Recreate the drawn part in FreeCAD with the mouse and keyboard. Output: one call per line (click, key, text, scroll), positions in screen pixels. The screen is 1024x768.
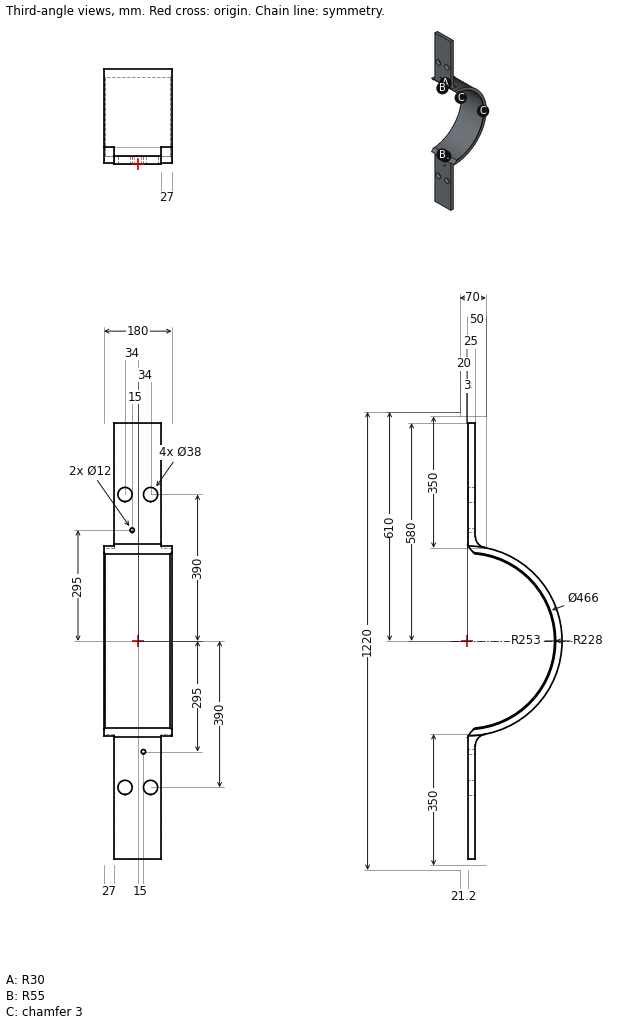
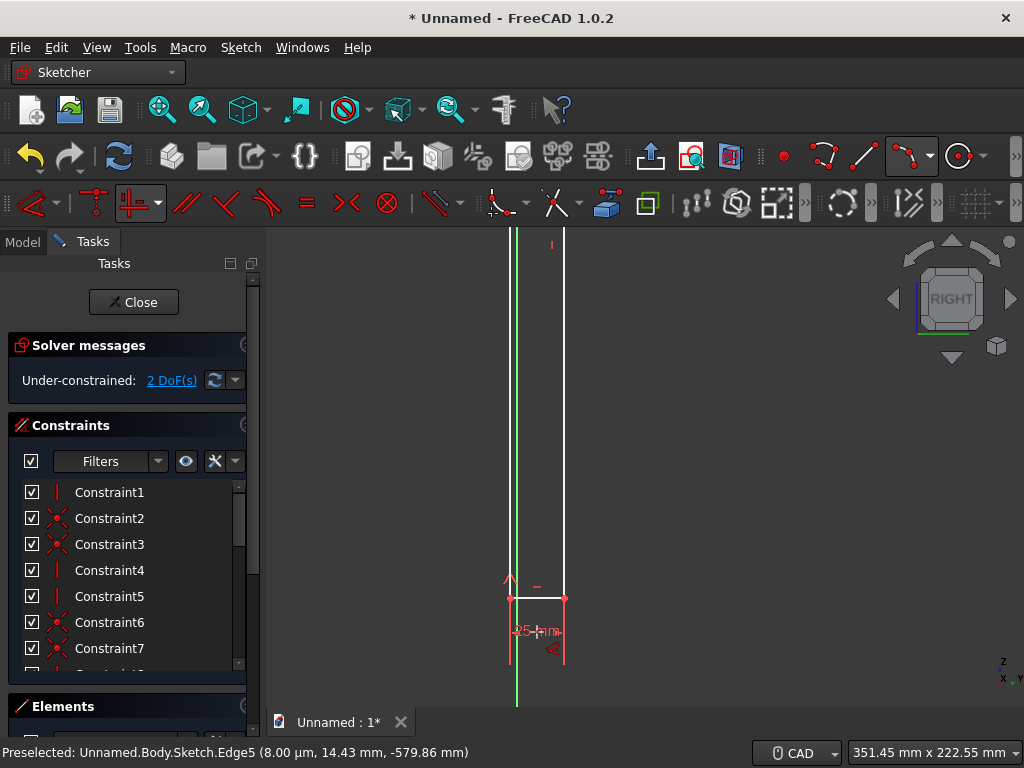
scroll(550, 606, down, 11)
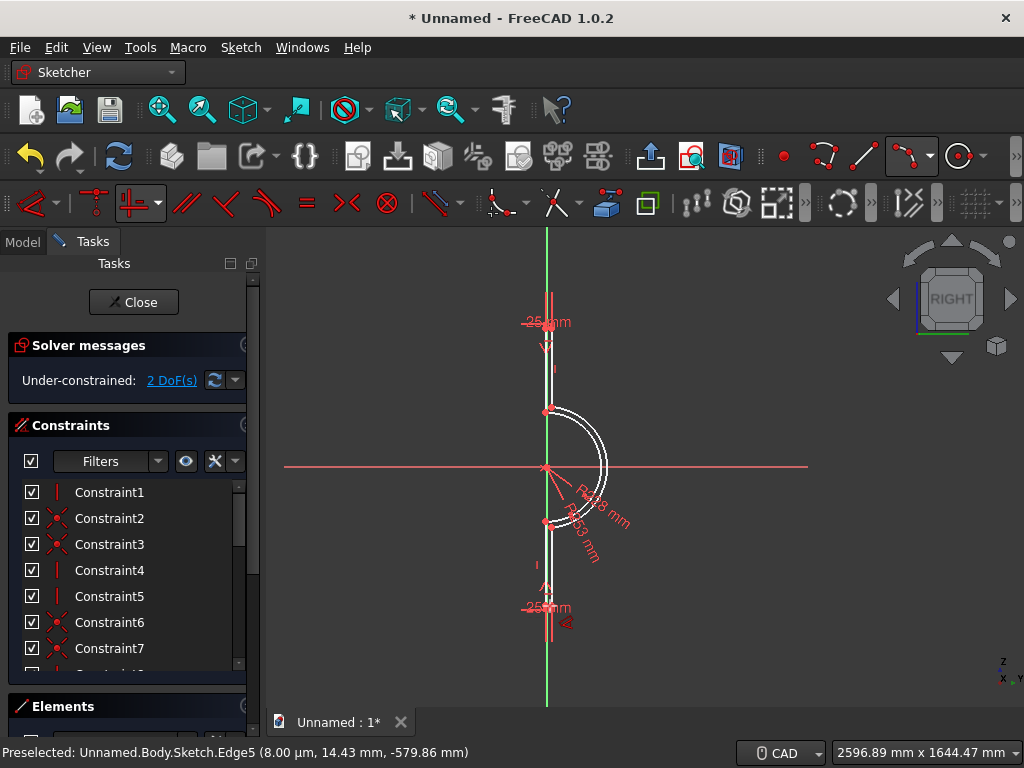
scroll(546, 329, up, 21)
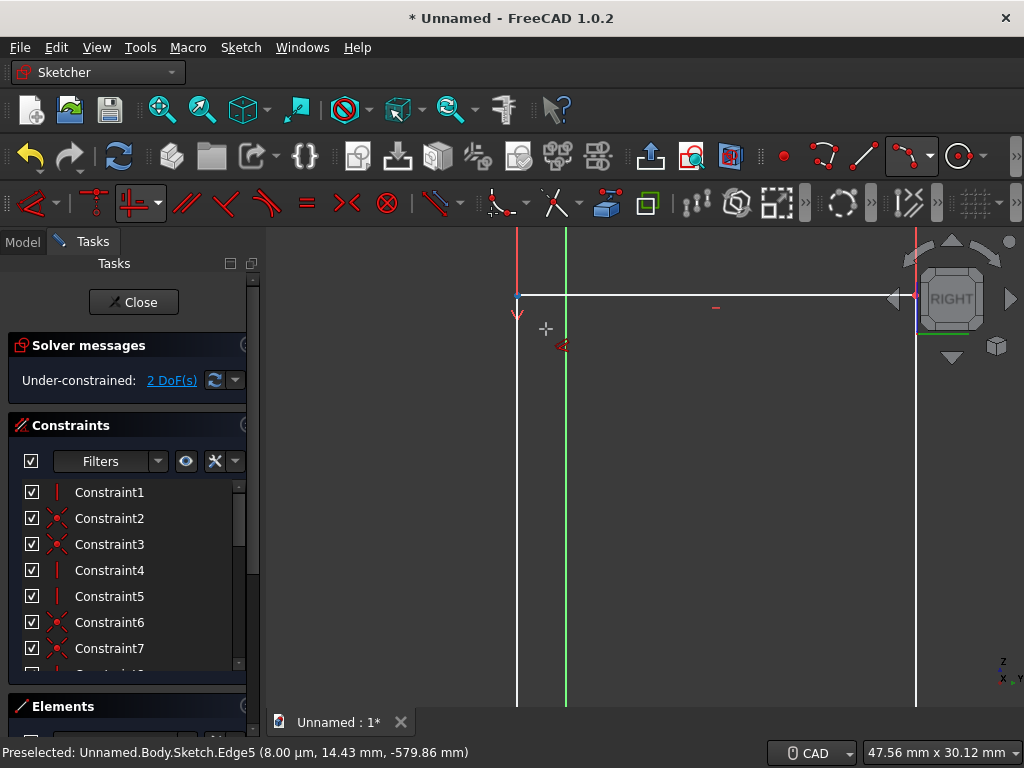
click(517, 295)
click(542, 261)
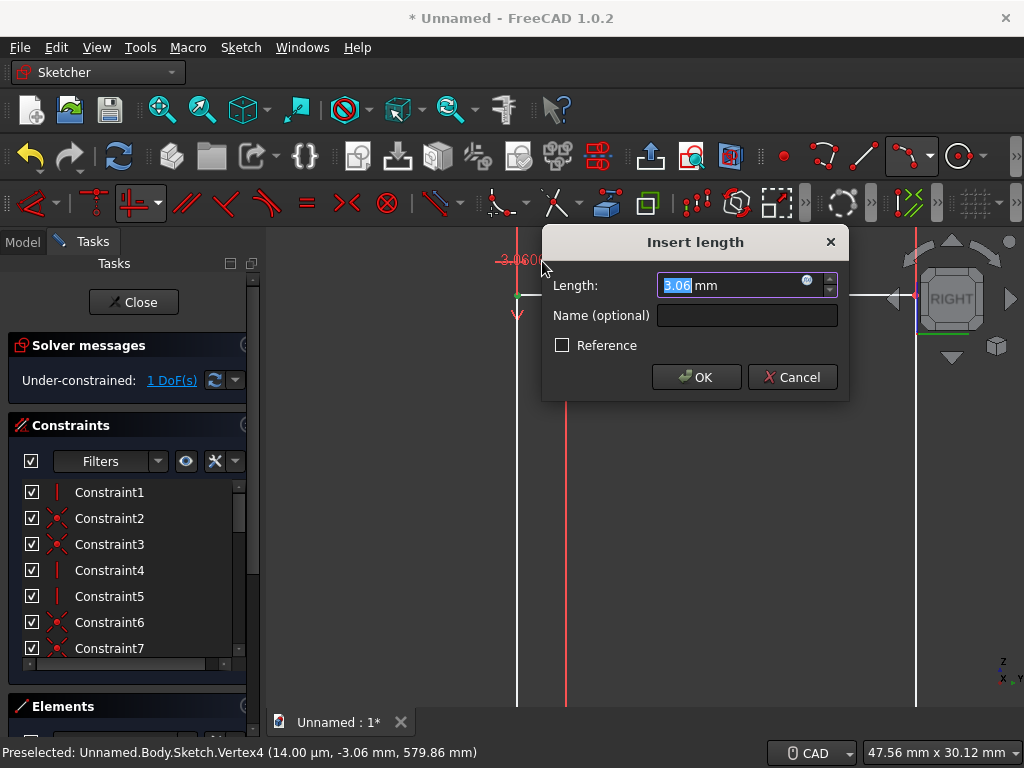
text(3)
key(Return)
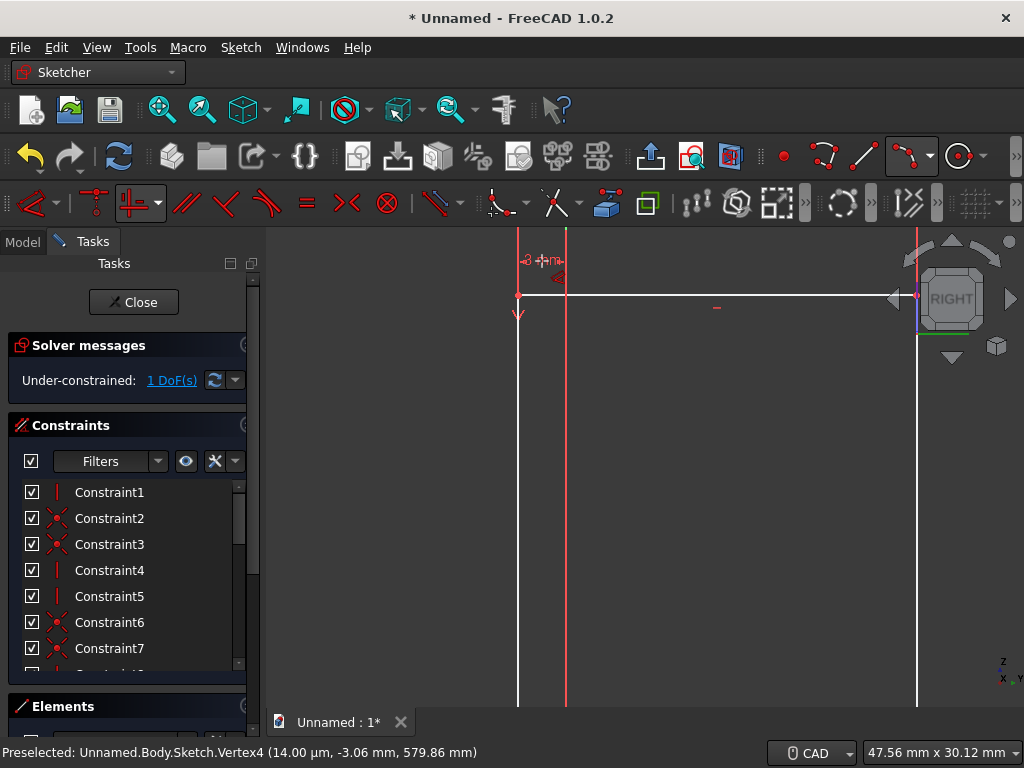
scroll(576, 467, down, 15)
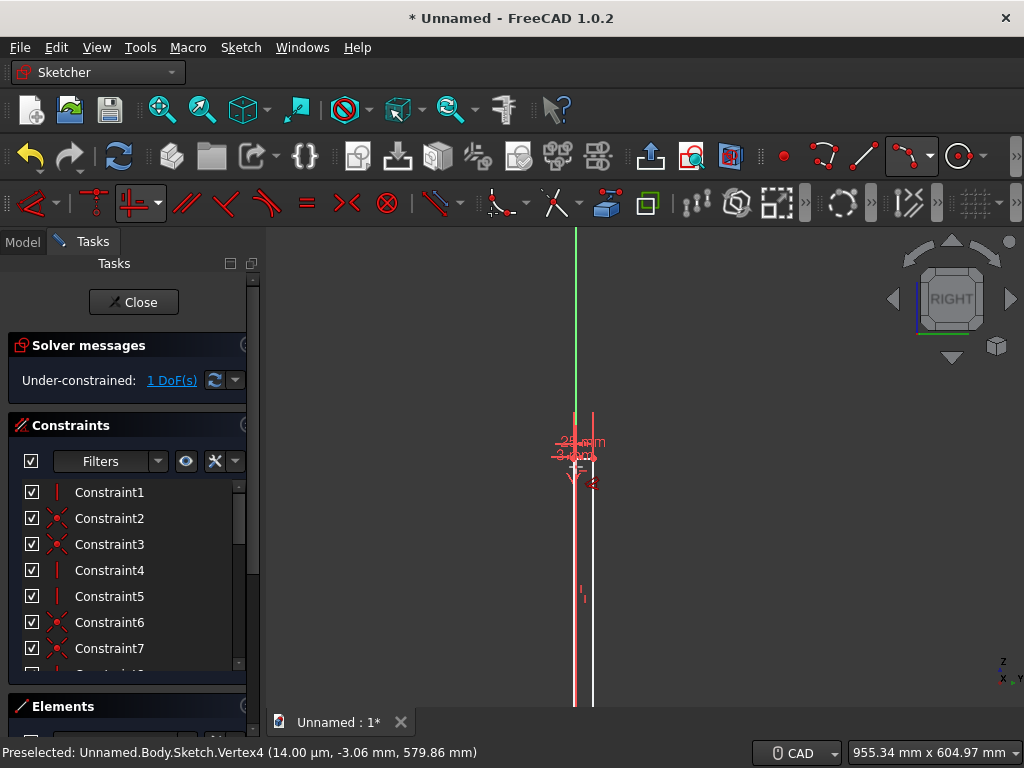
scroll(534, 272, down, 6)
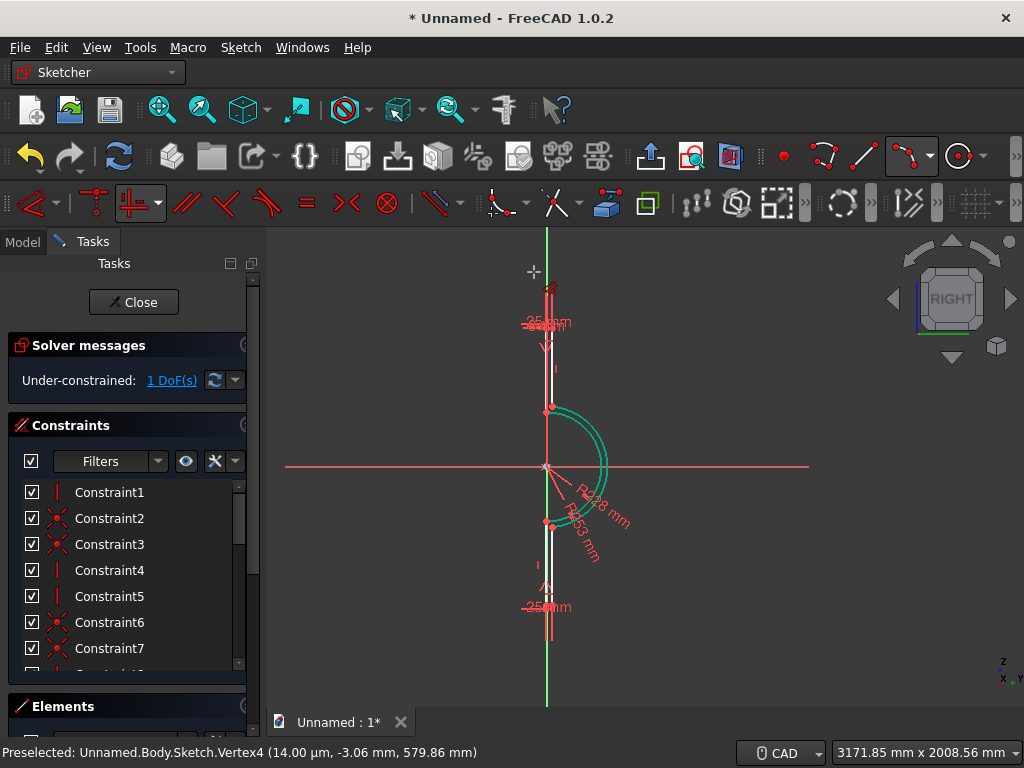
scroll(552, 328, up, 4)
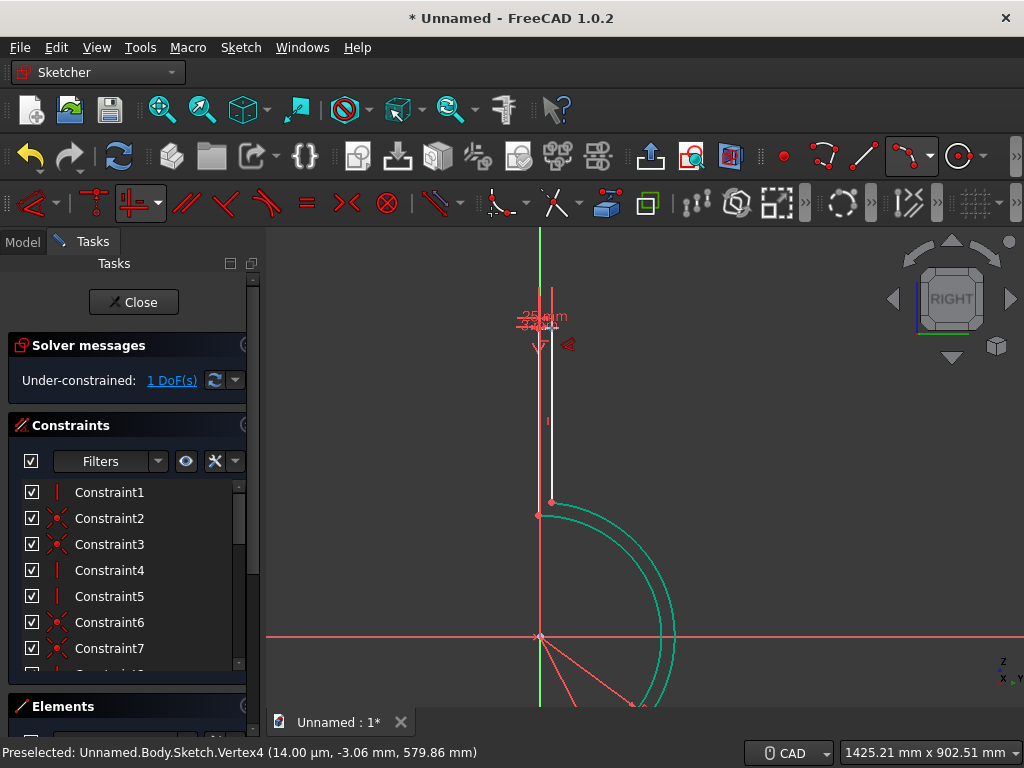
click(552, 329)
click(506, 483)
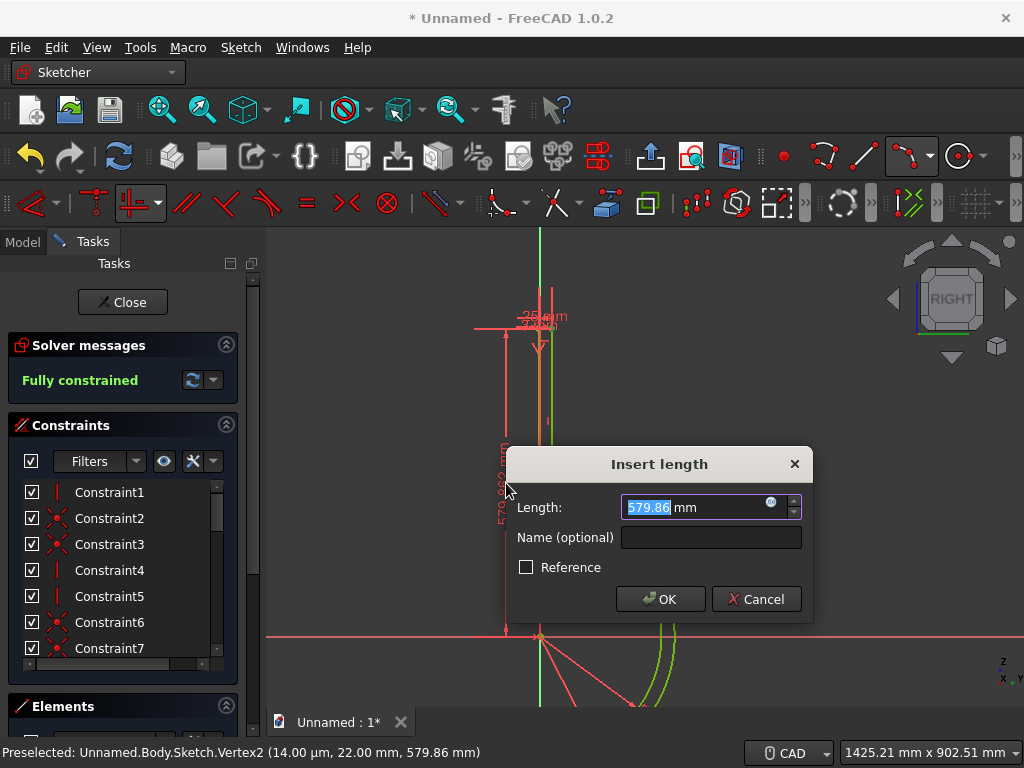
text(580)
key(Return)
key(Escape)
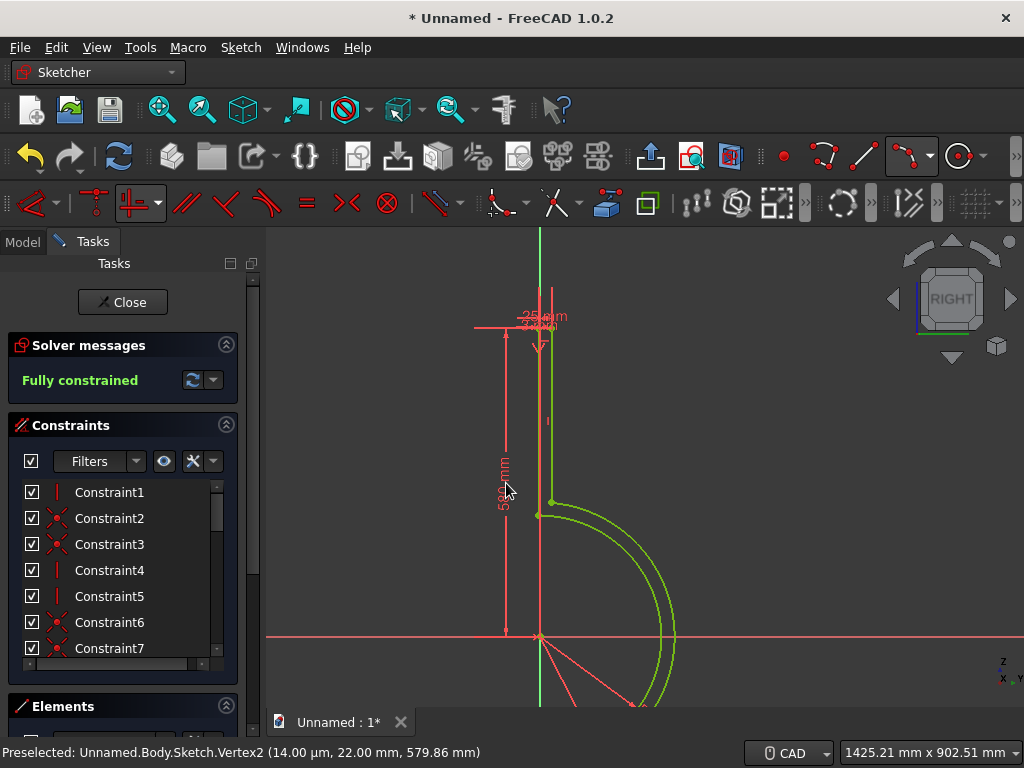
click(123, 302)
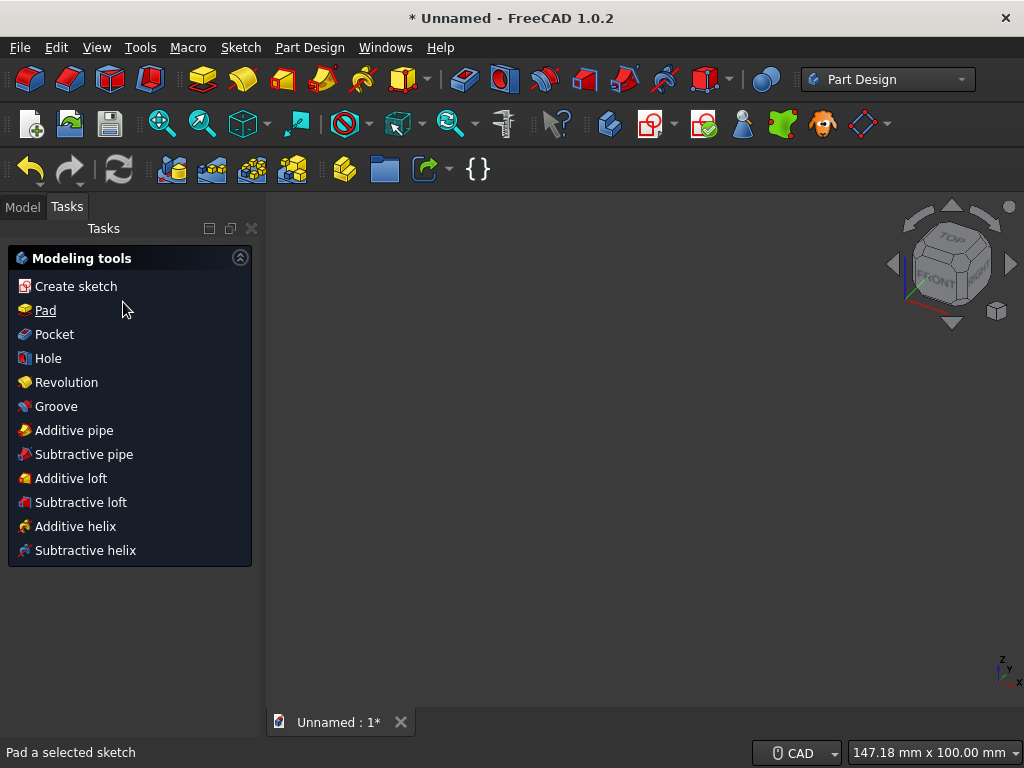
click(204, 80)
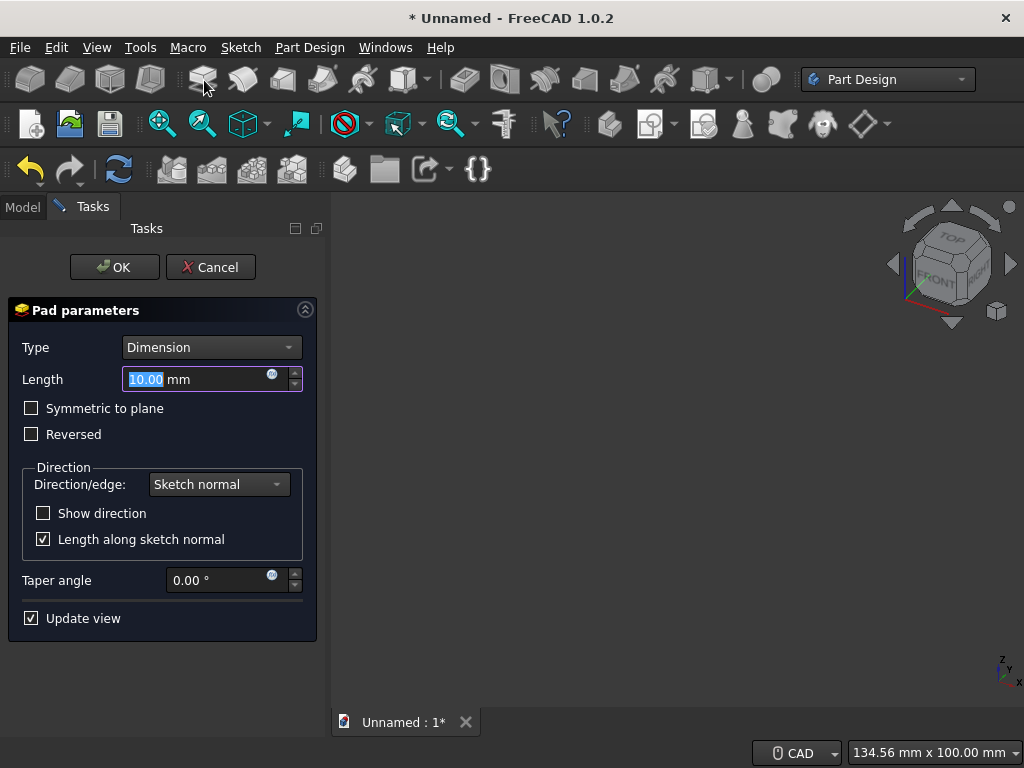
text(180)
key(Tab)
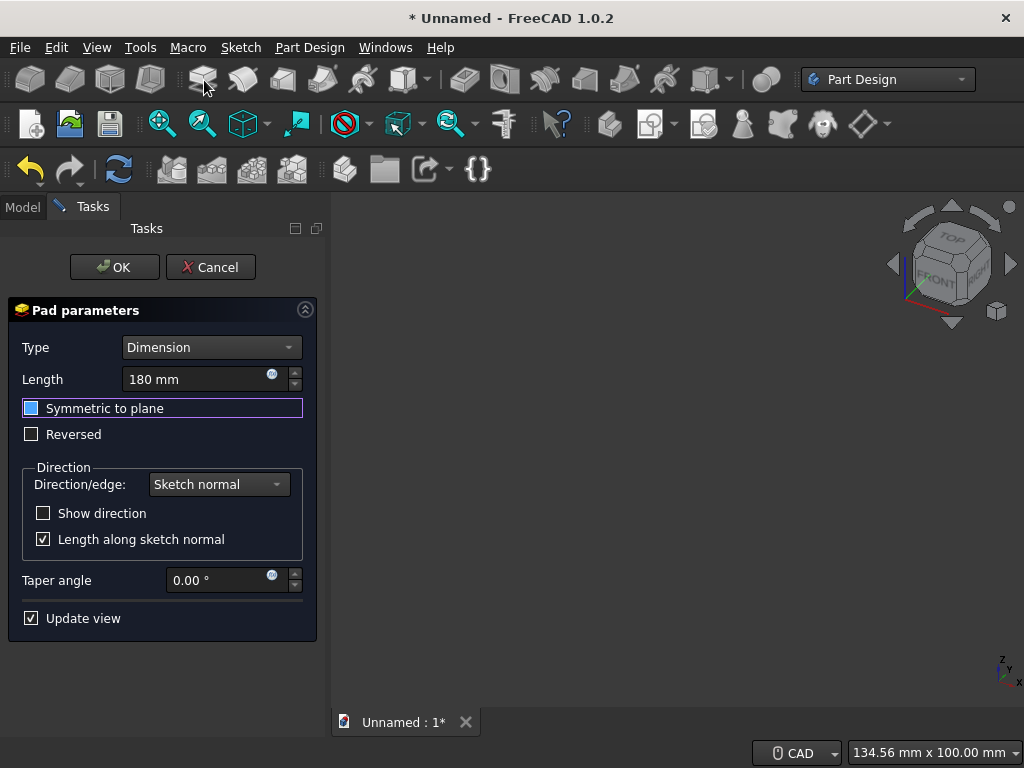
click(30, 408)